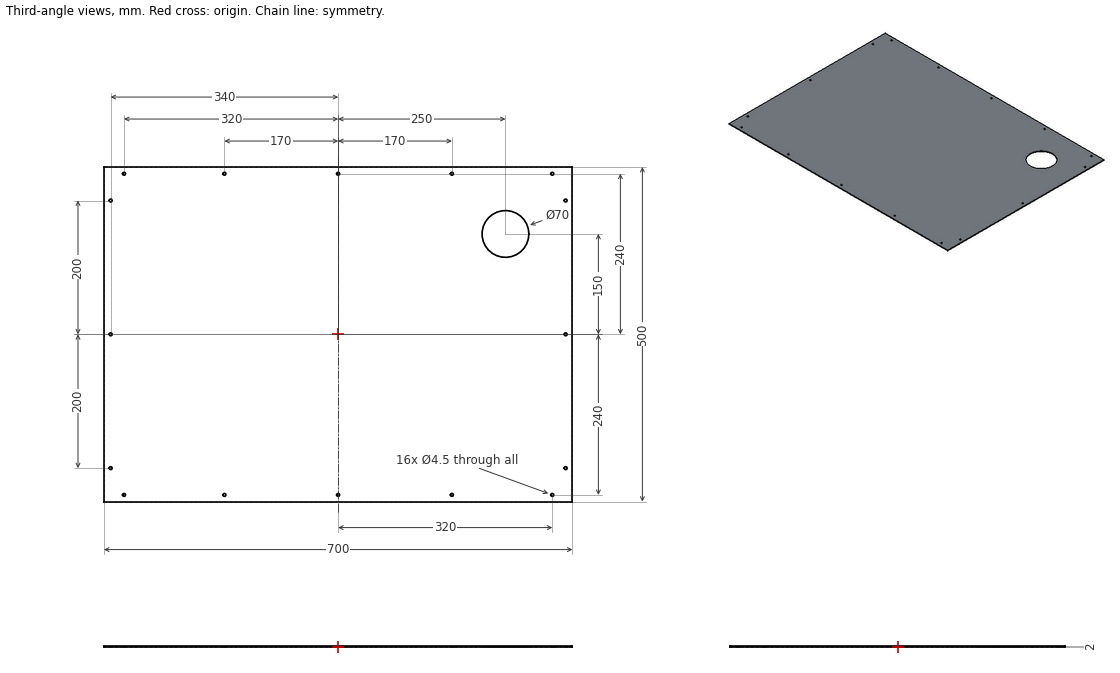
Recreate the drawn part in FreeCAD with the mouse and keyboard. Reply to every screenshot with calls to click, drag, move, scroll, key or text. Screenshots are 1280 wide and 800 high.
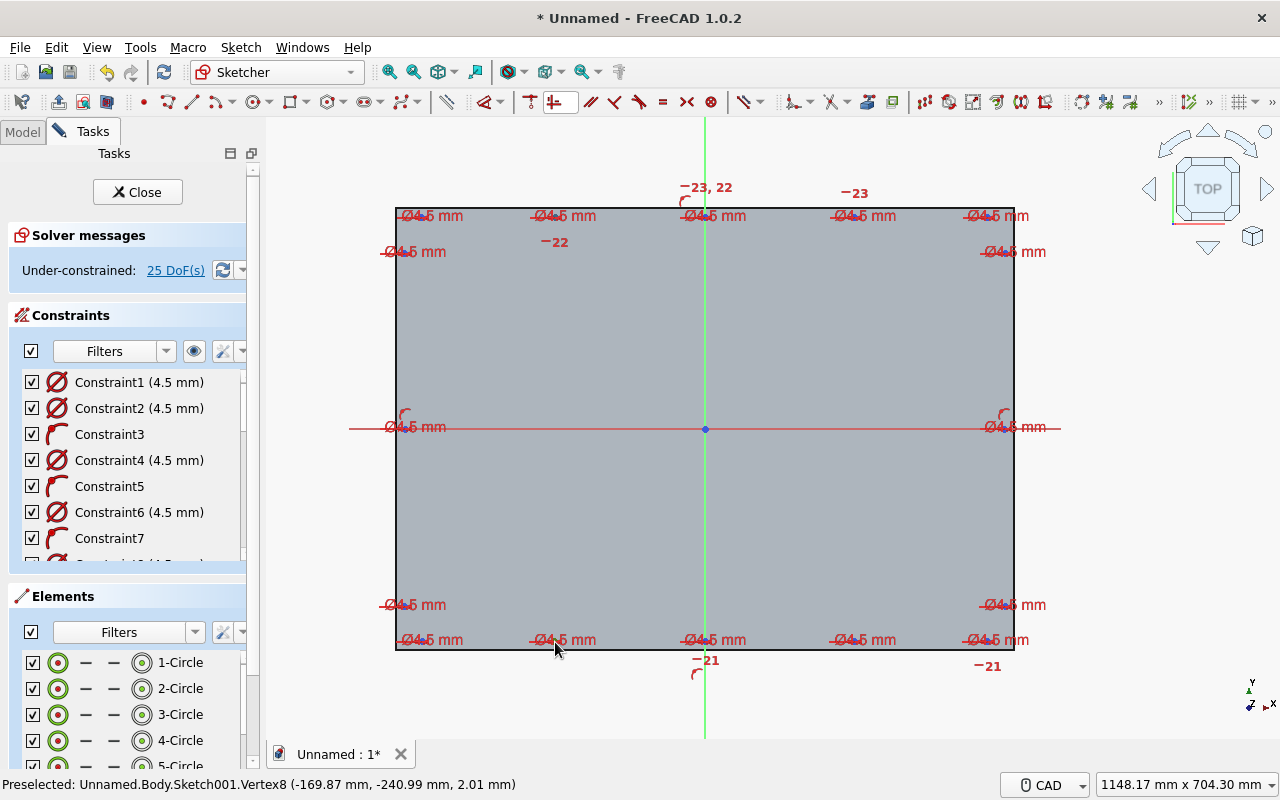
key(v)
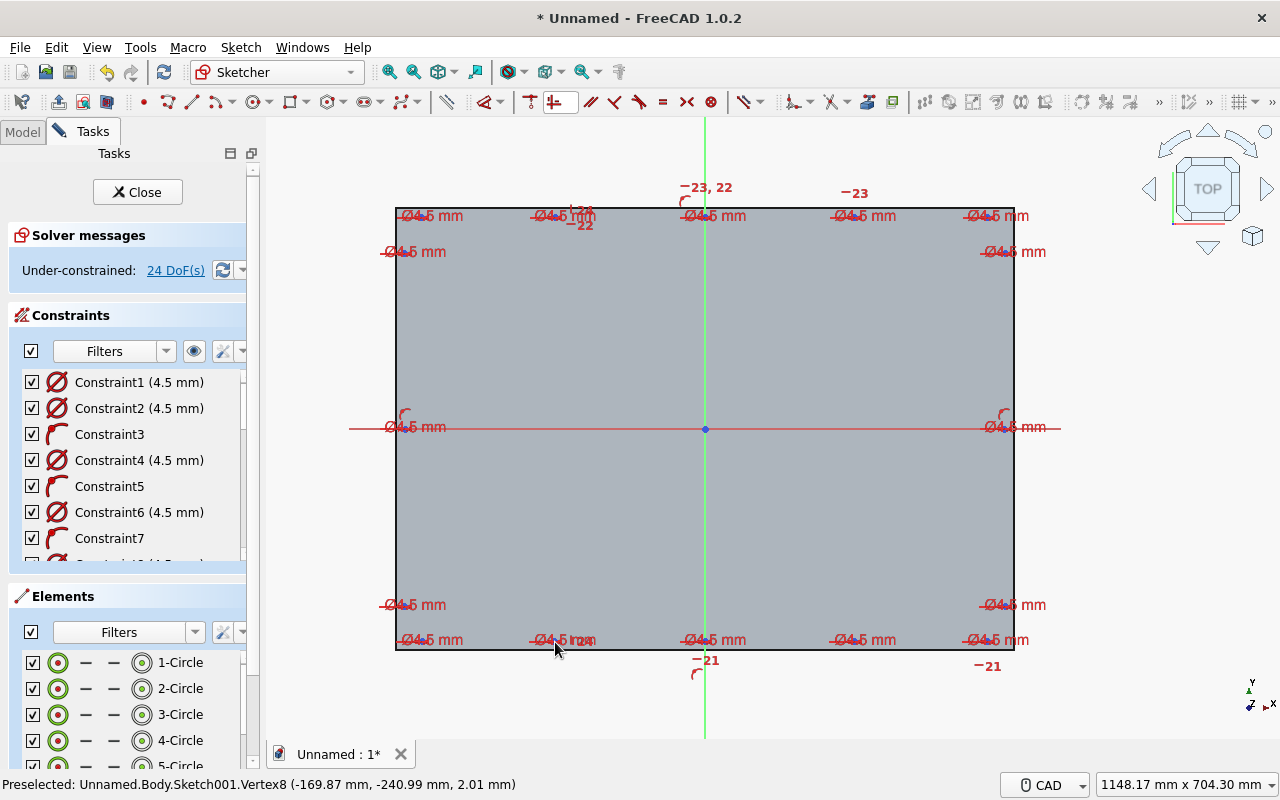
click(705, 642)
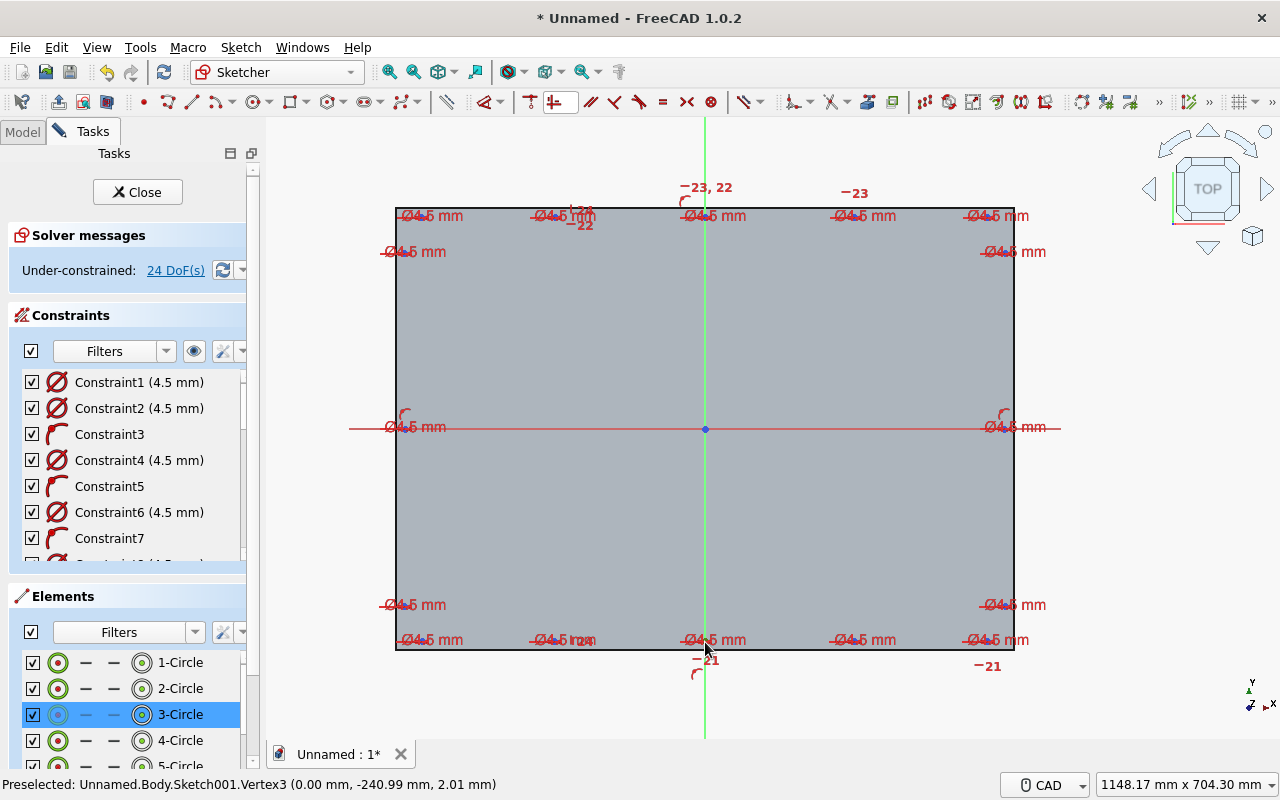
click(555, 642)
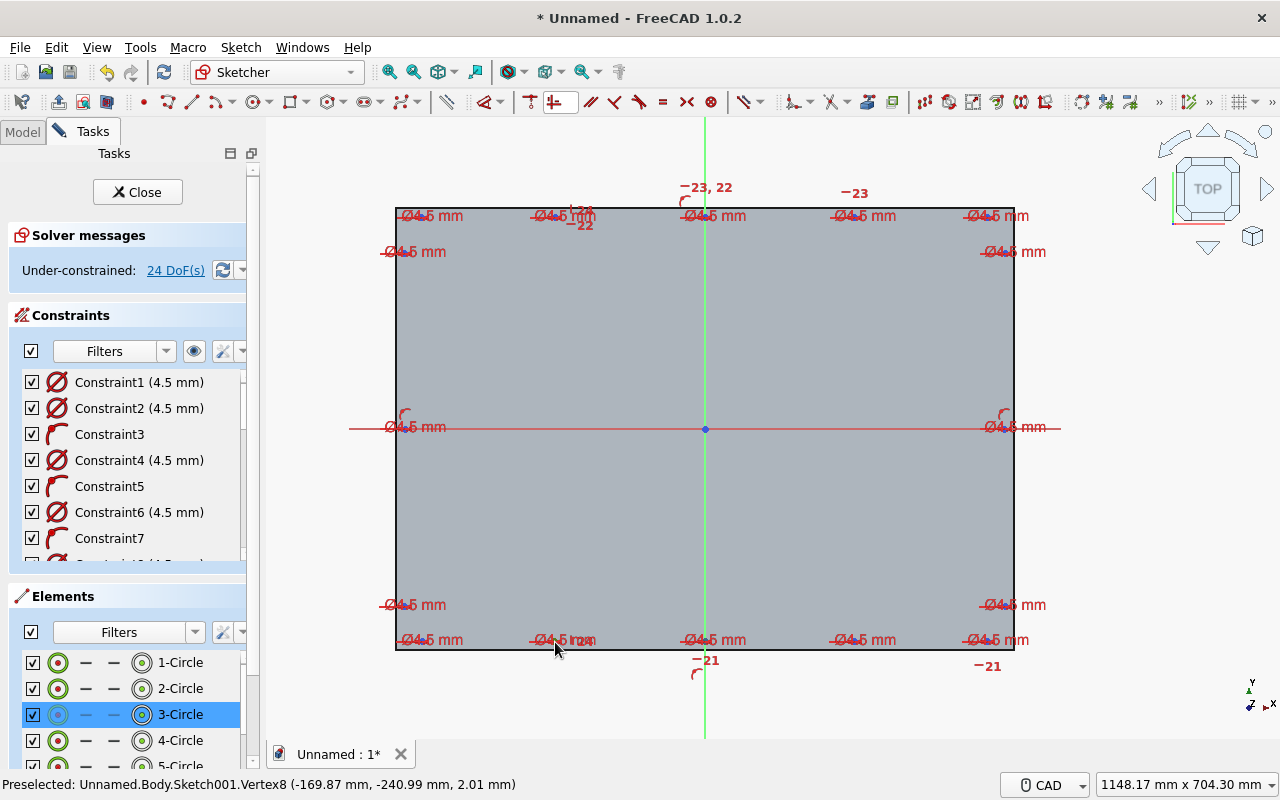
key(h)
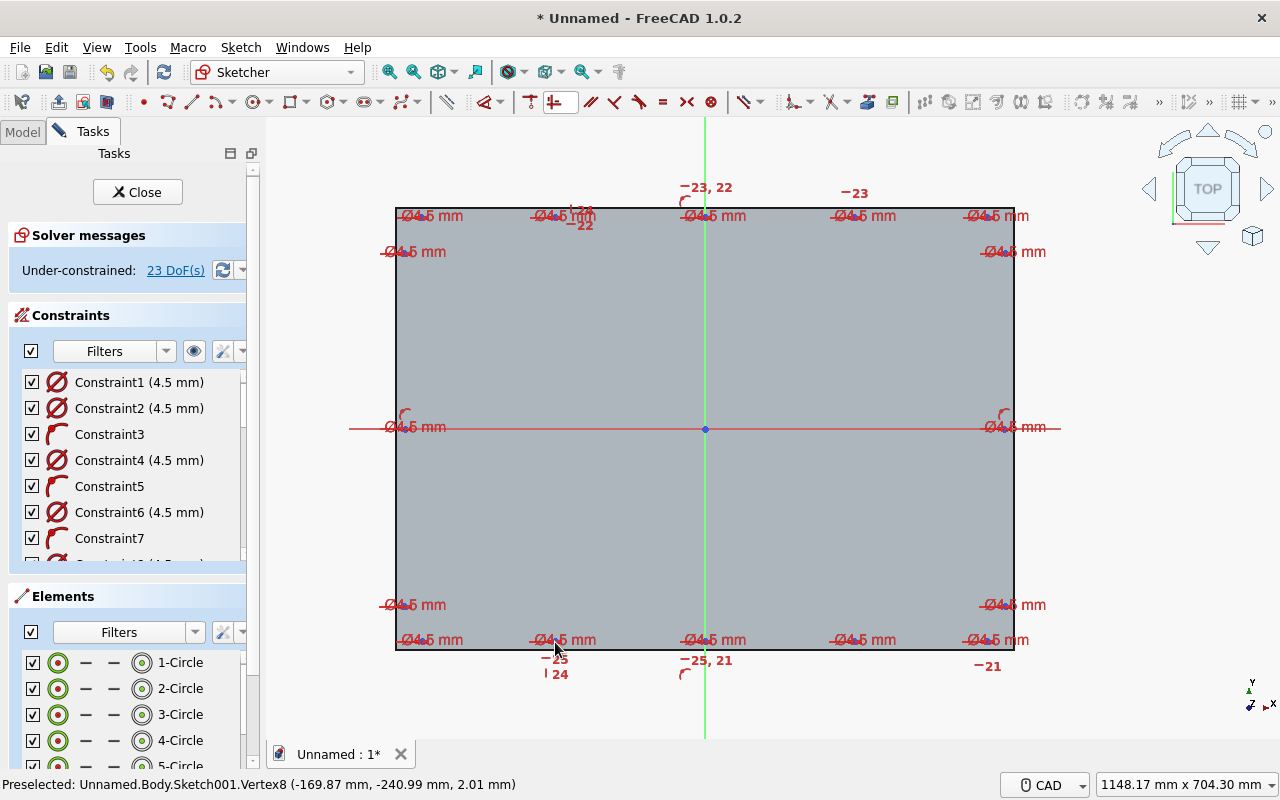
click(855, 218)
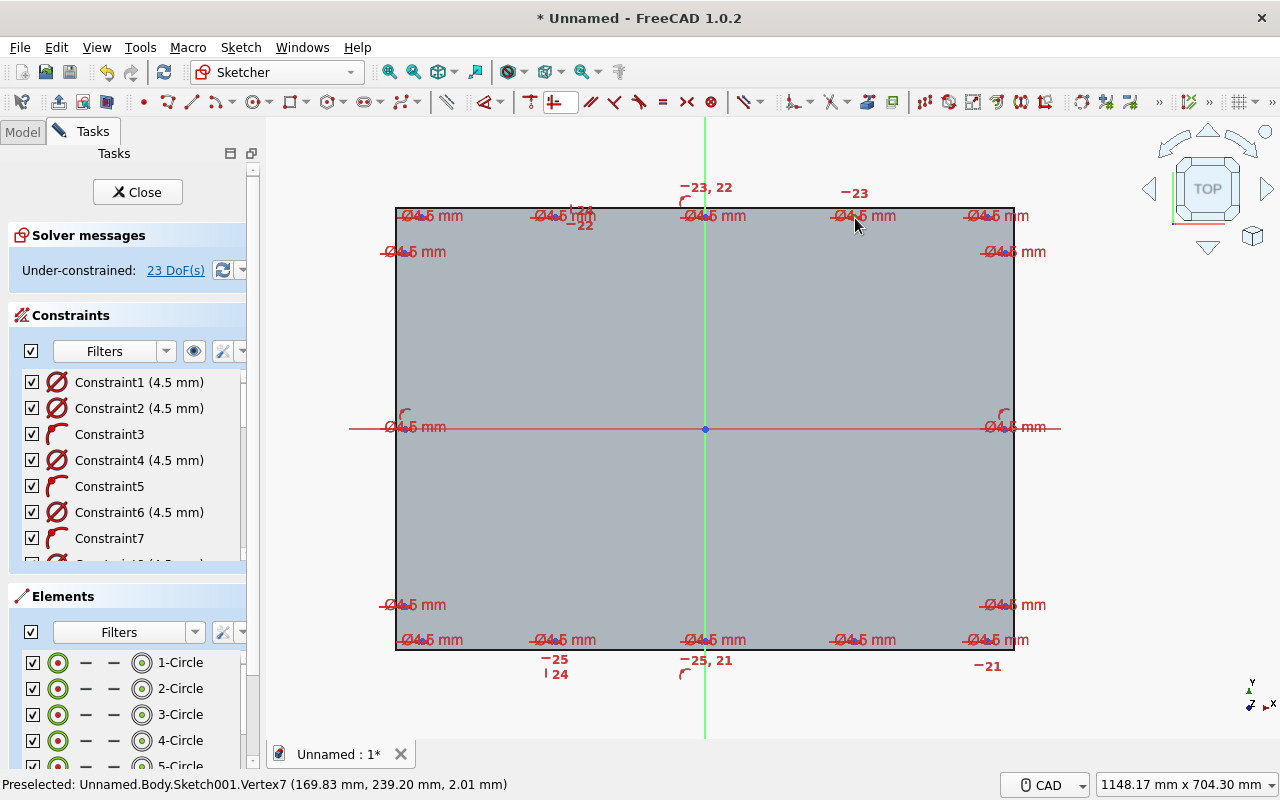
click(855, 642)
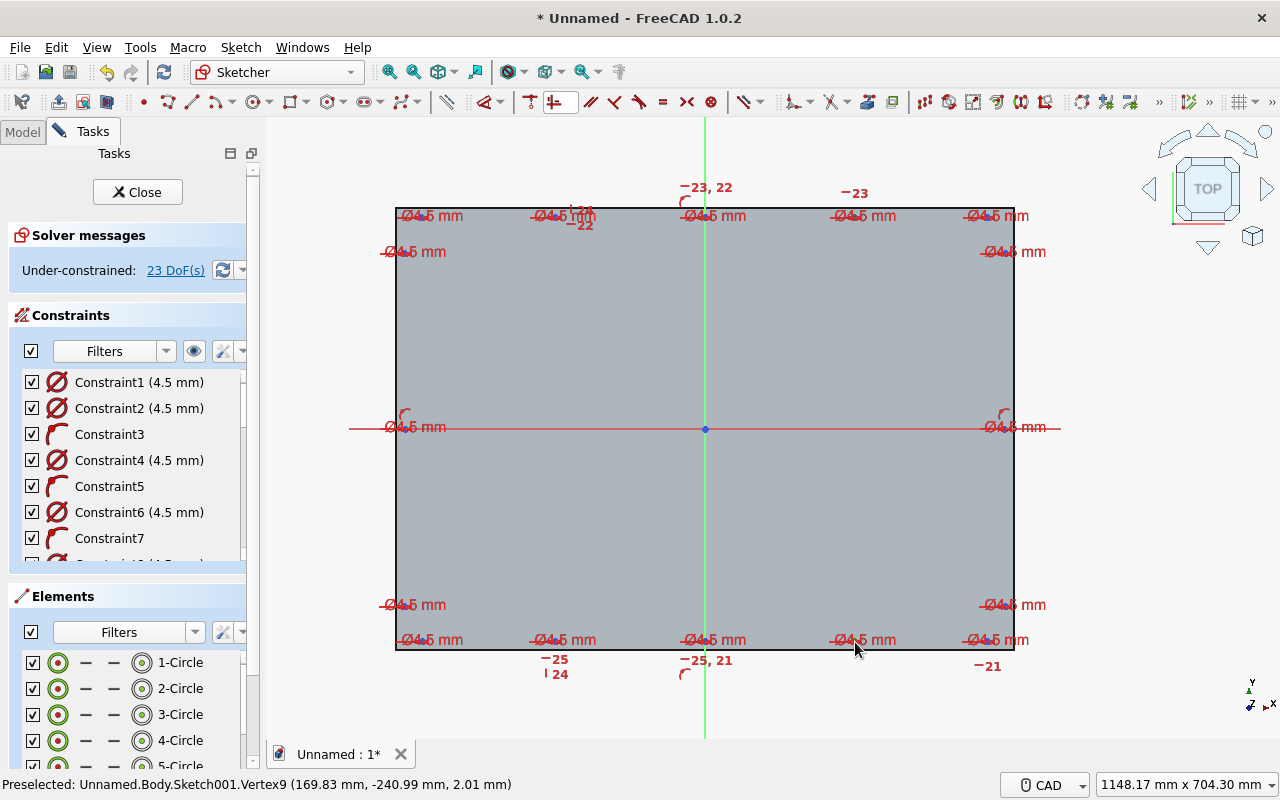
key(v)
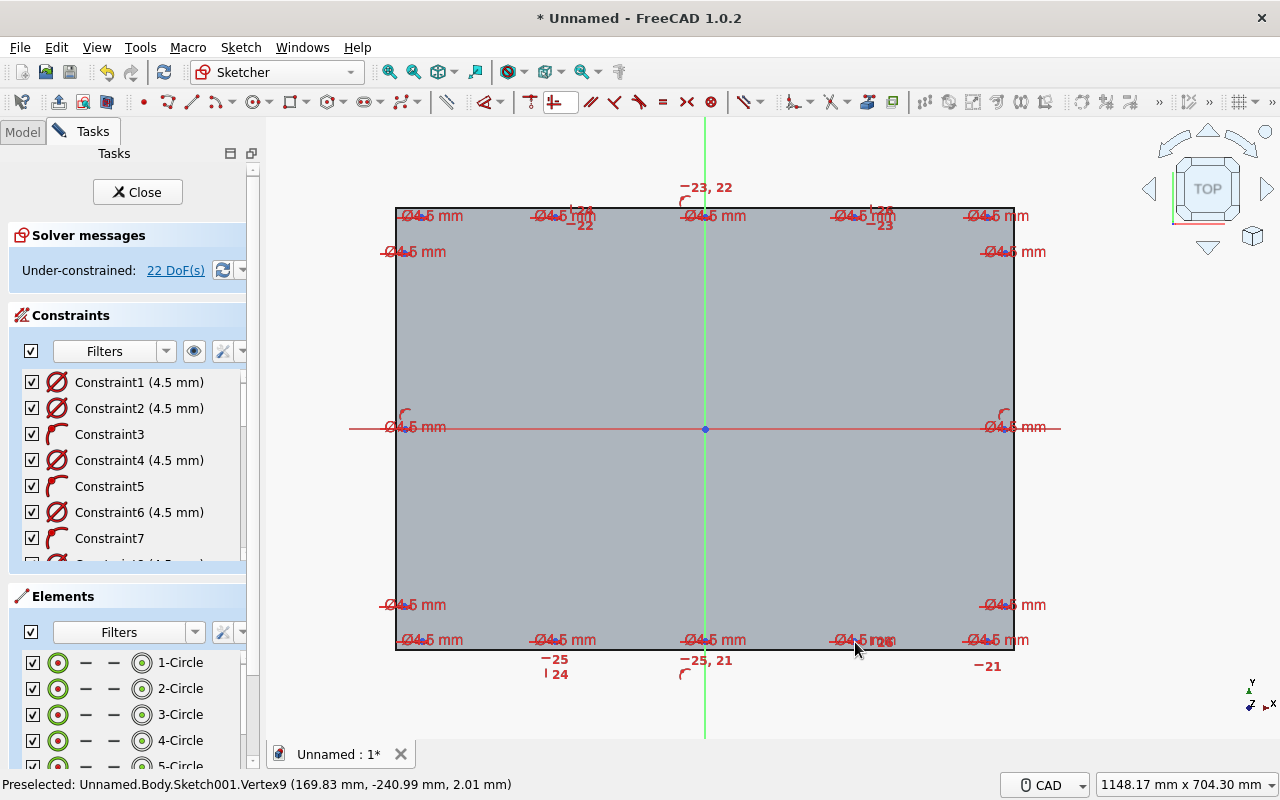
click(988, 642)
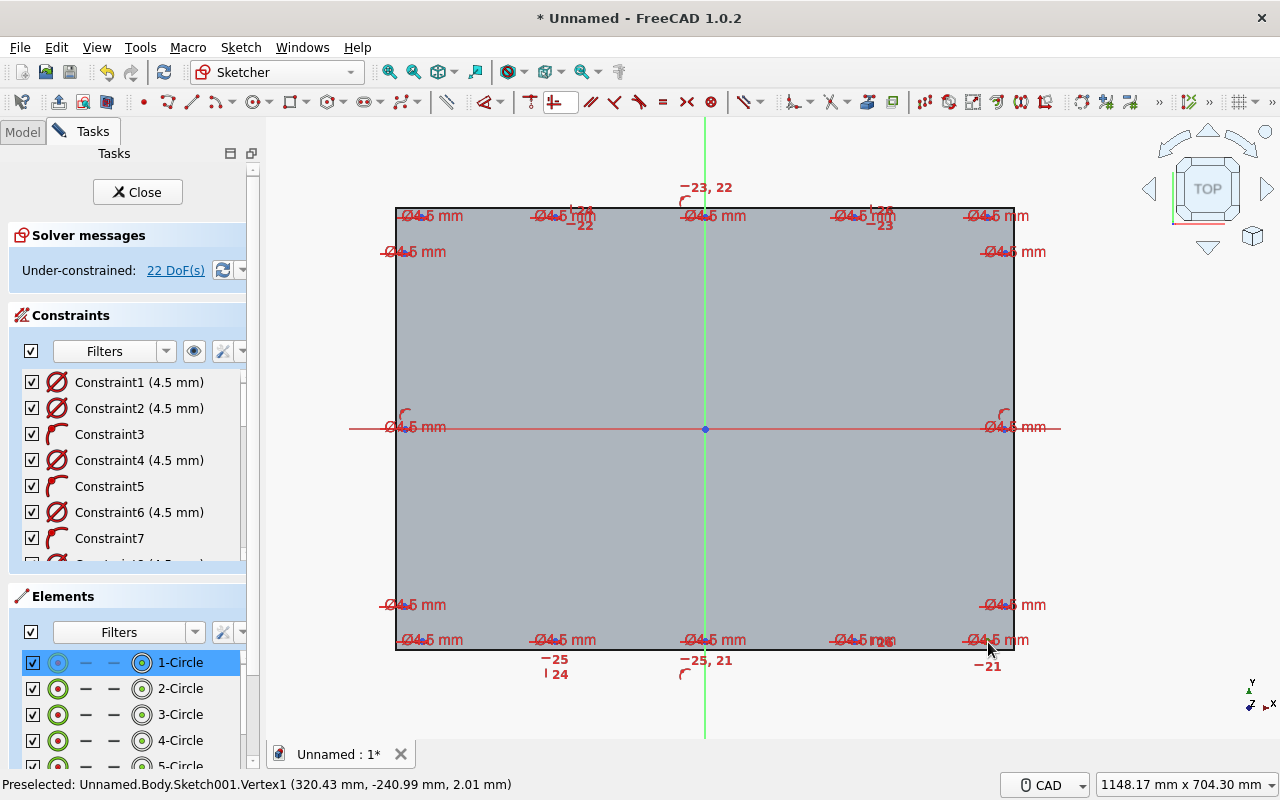
click(855, 642)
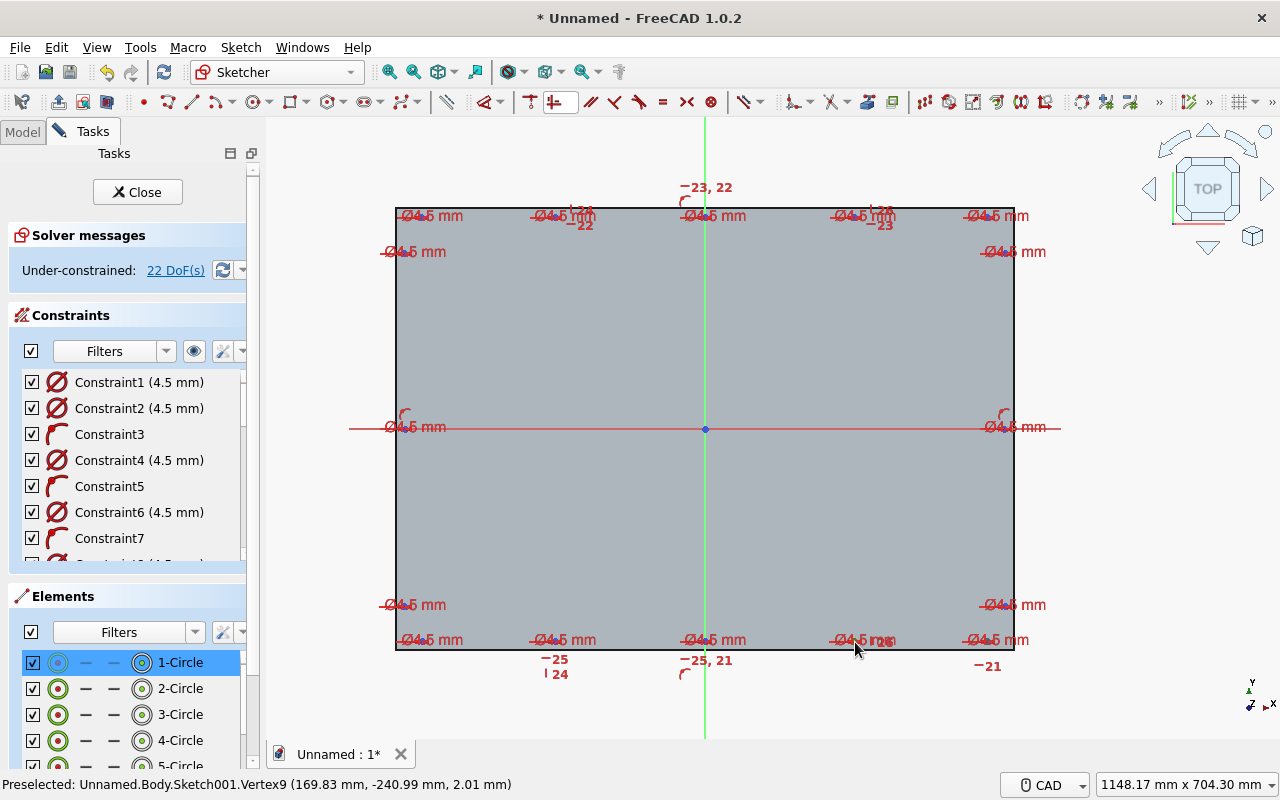
key(h)